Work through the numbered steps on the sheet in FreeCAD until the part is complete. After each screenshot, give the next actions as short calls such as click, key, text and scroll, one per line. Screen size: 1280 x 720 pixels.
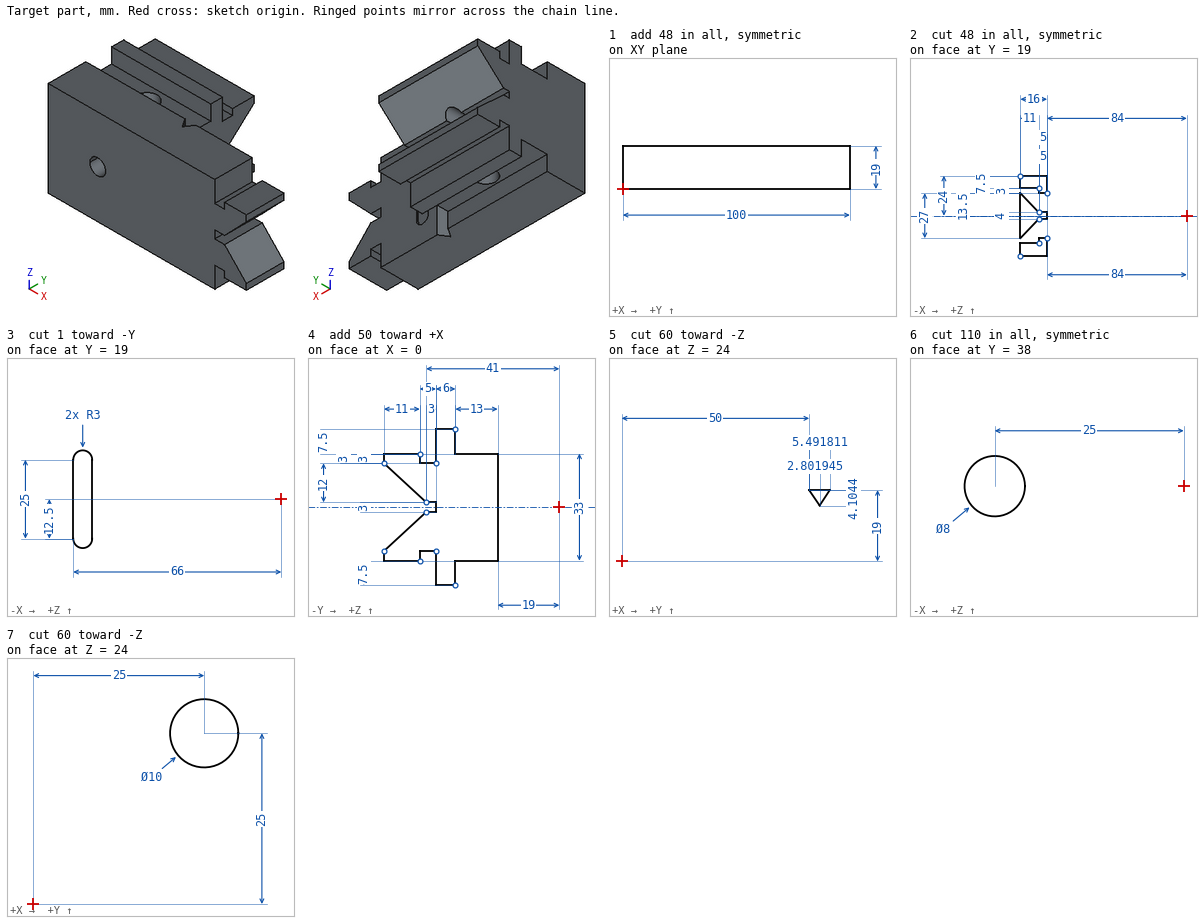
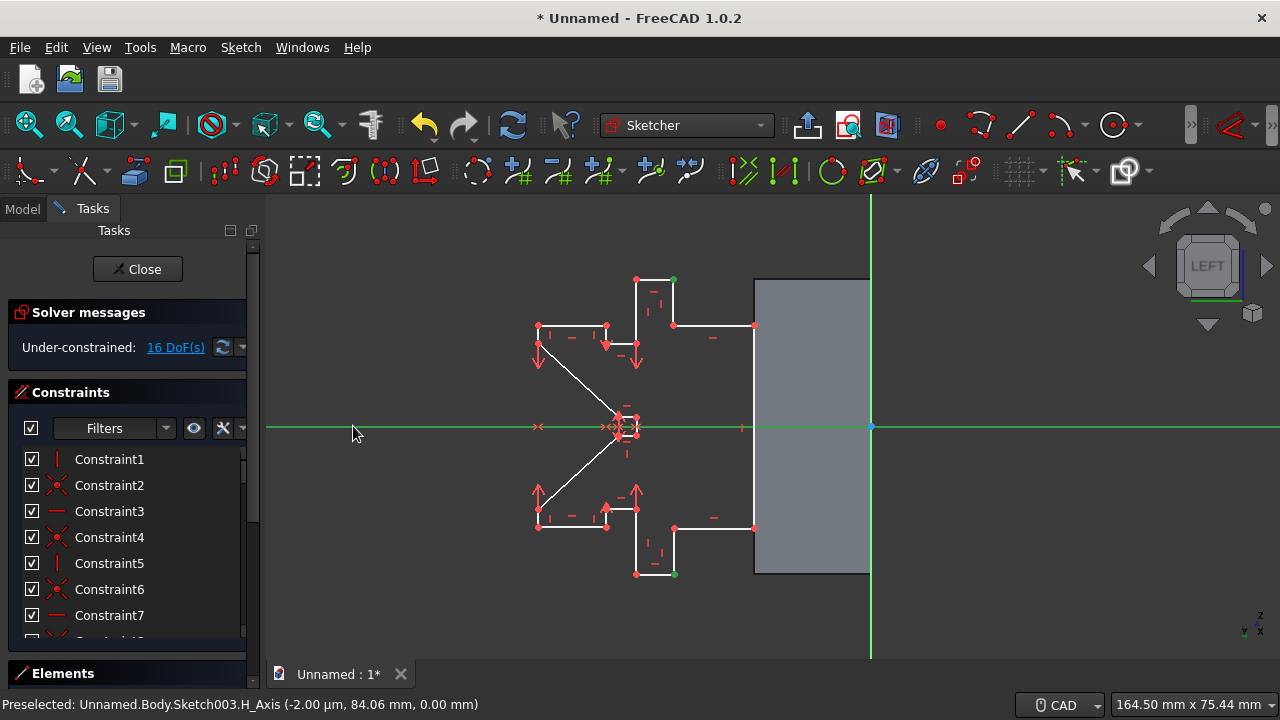
key(s)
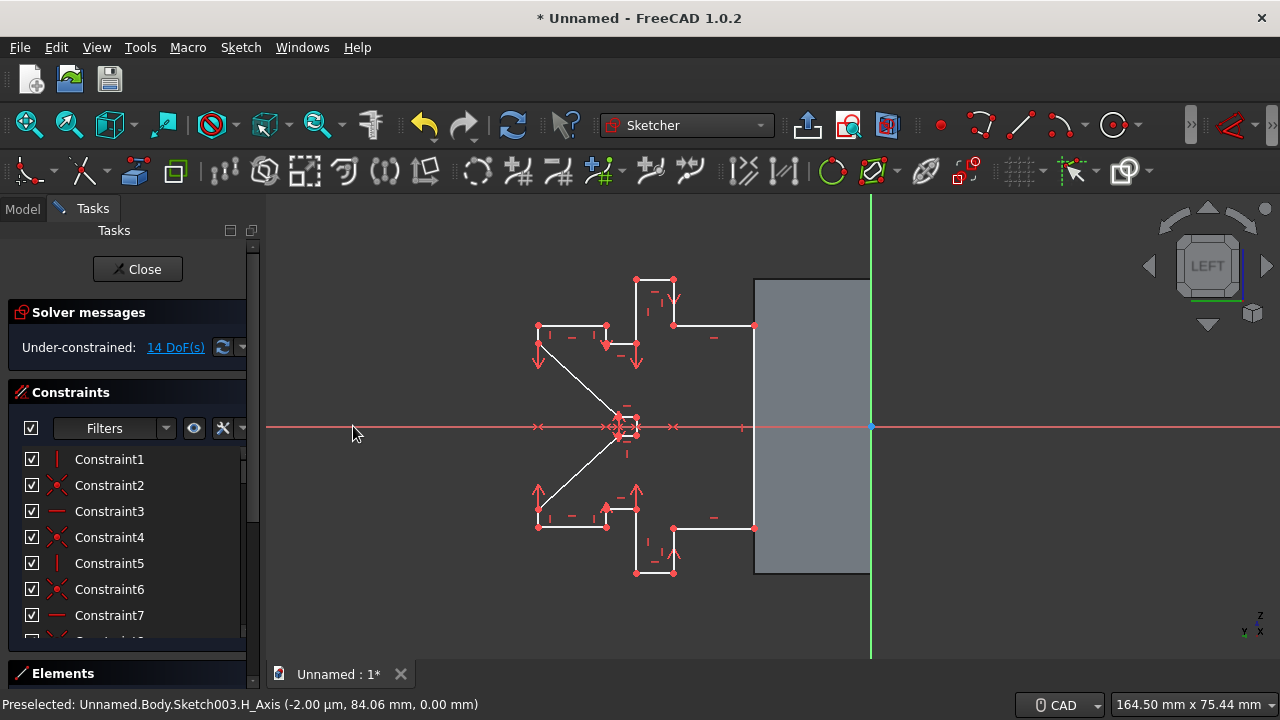
click(1230, 126)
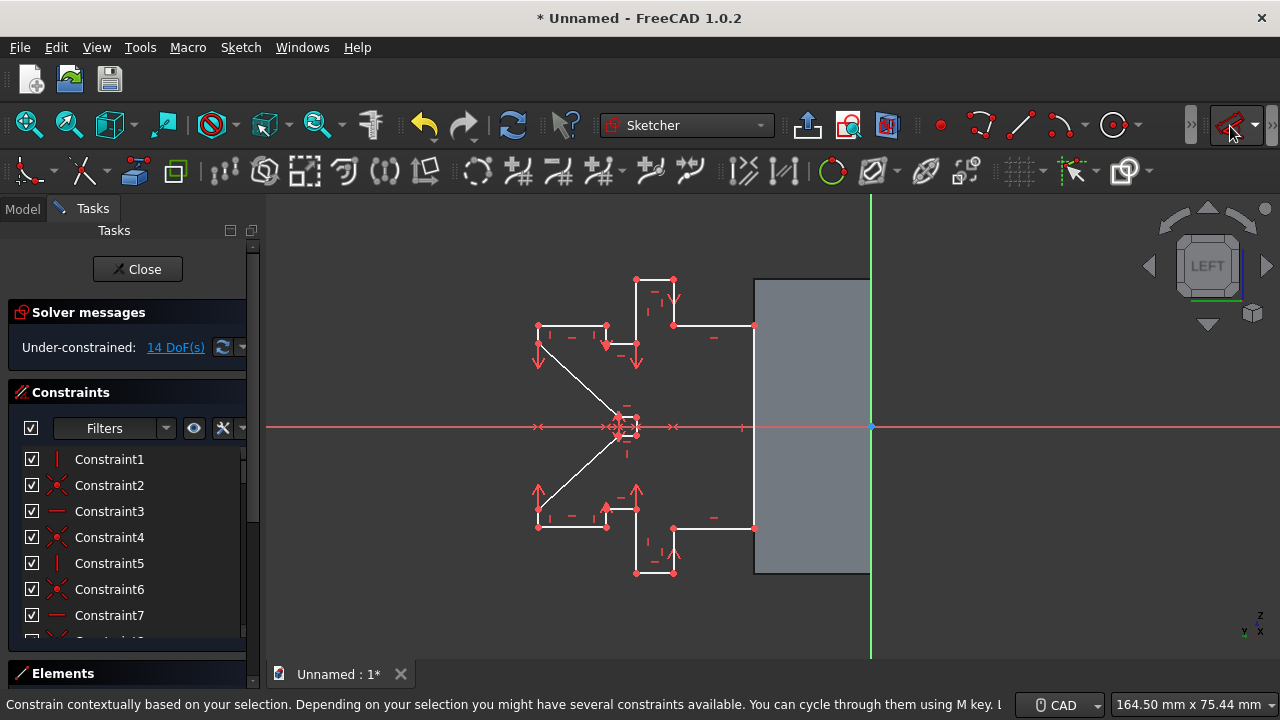
scroll(663, 280, up, 2)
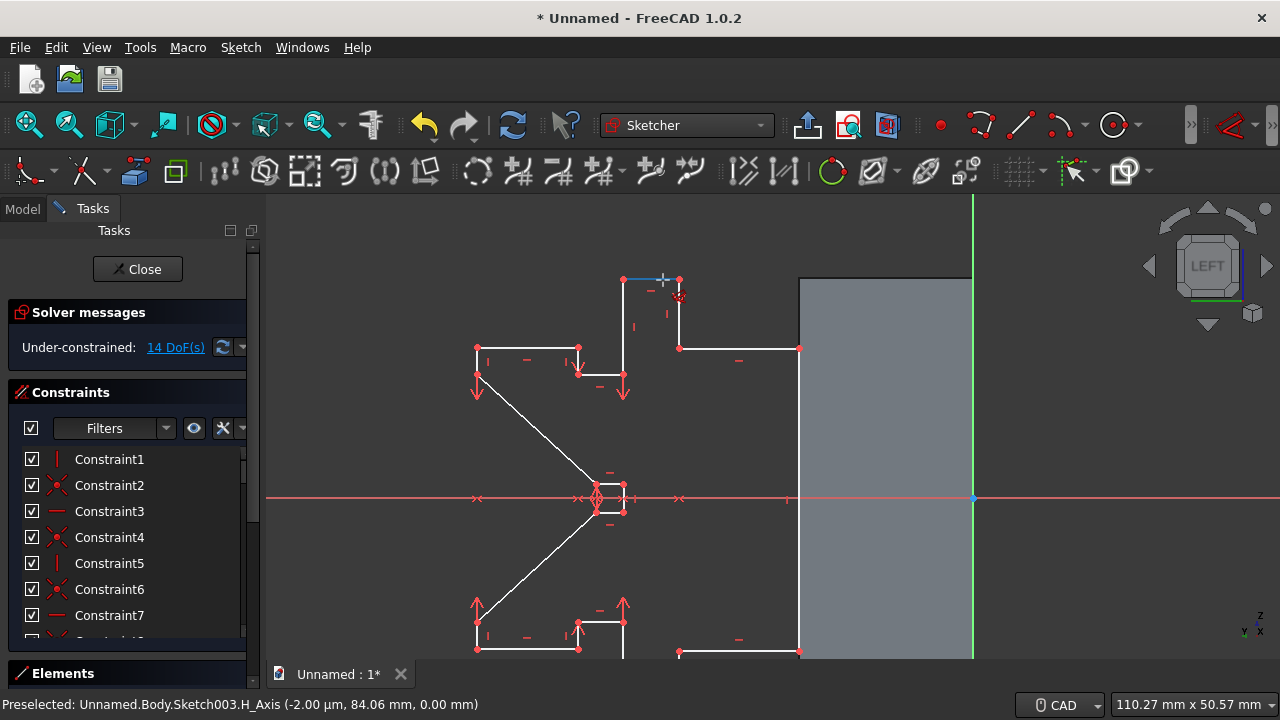
click(662, 279)
click(651, 245)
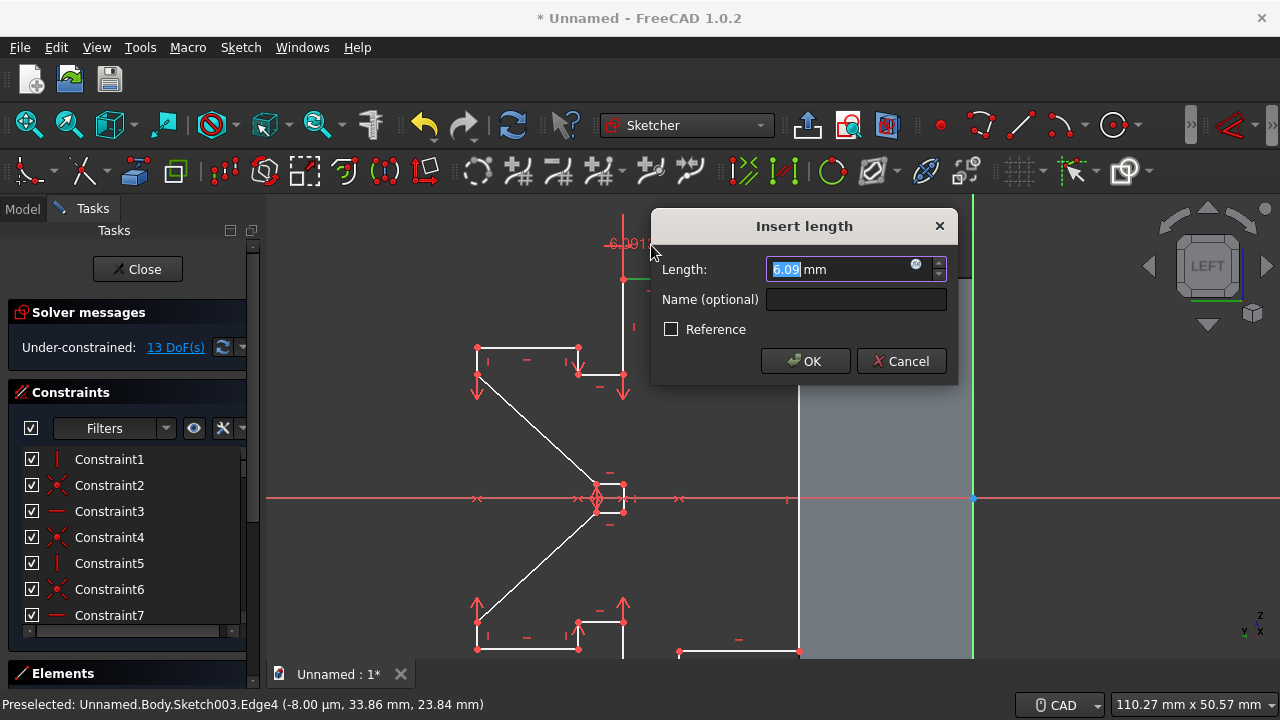
text(6)
key(Return)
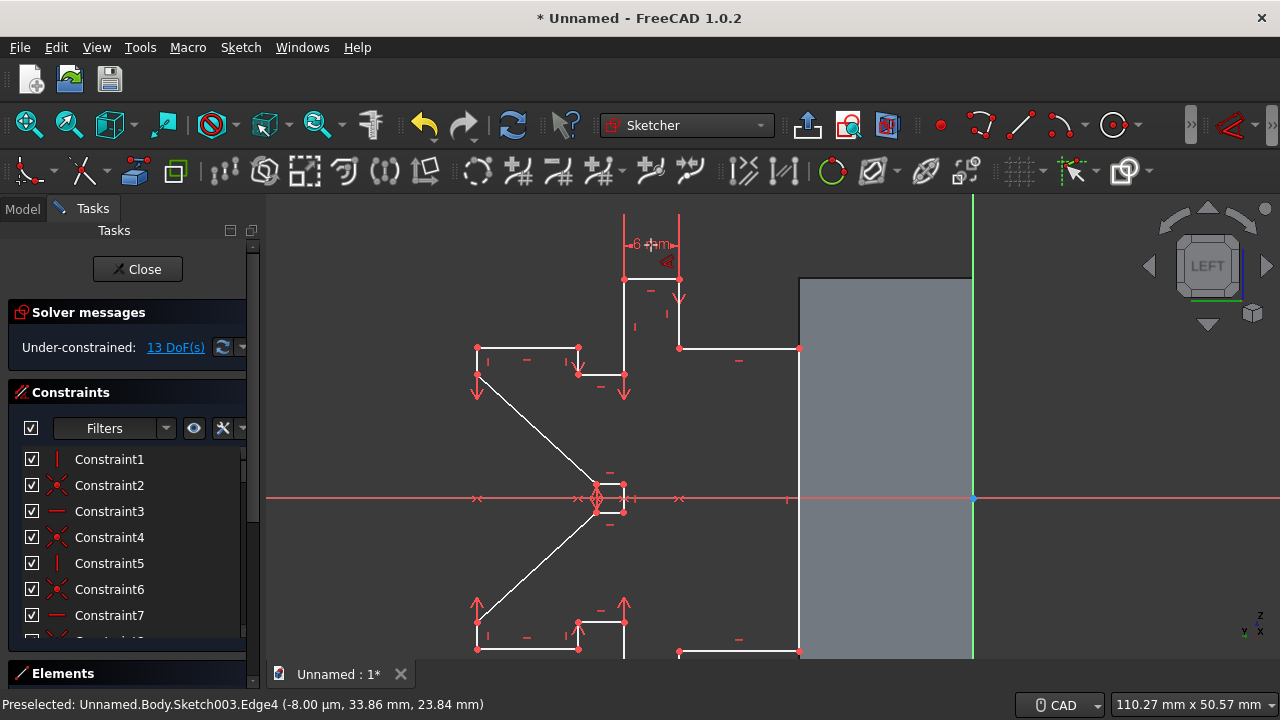
click(610, 375)
click(601, 341)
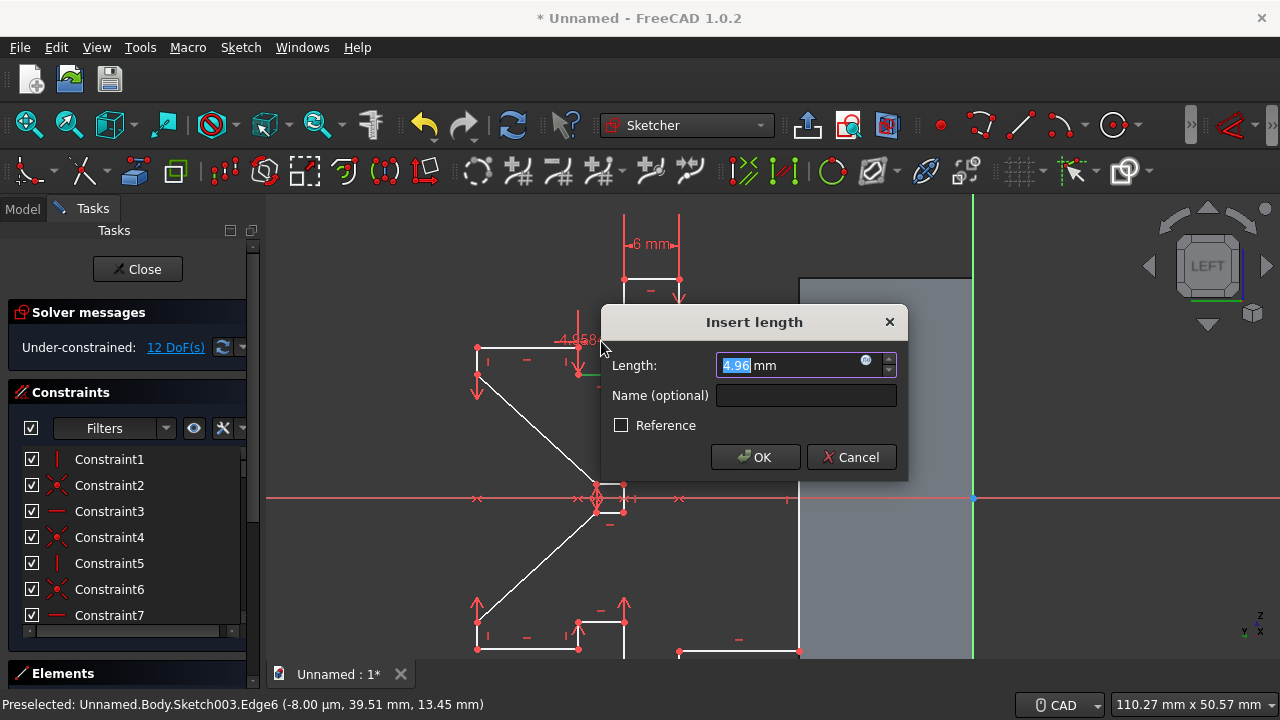
text(5)
key(Return)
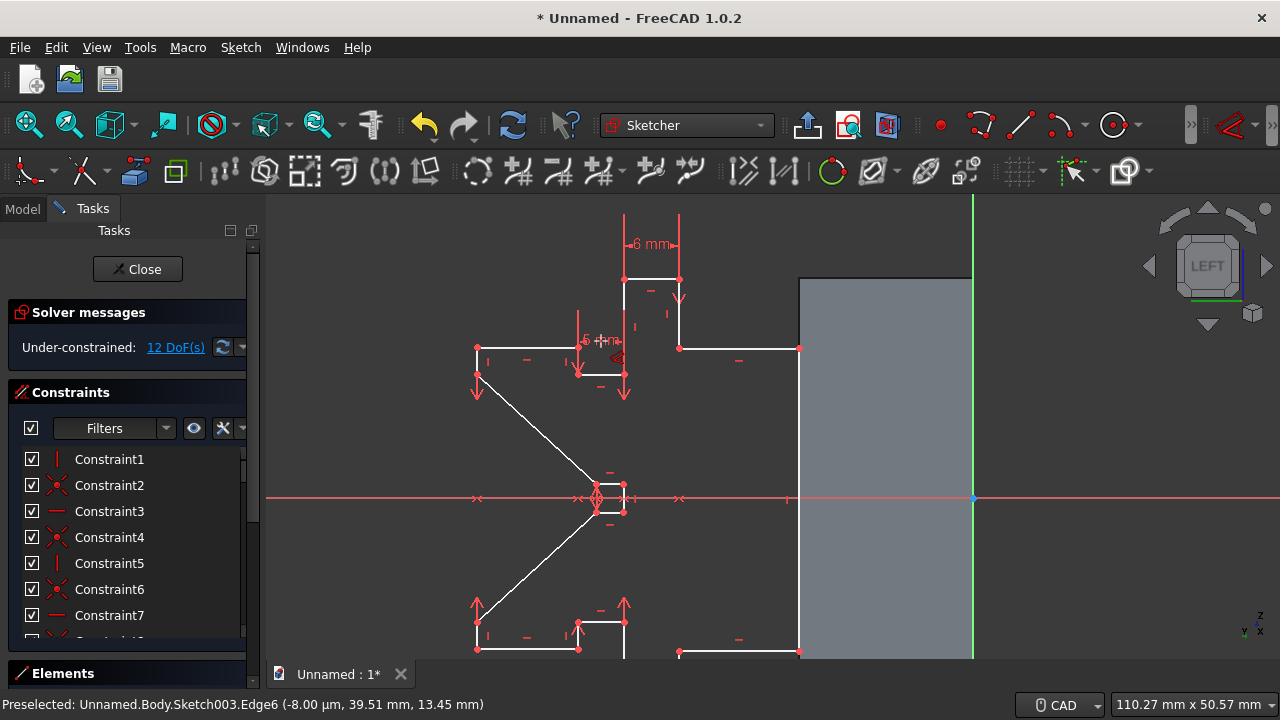
scroll(578, 364, up, 2)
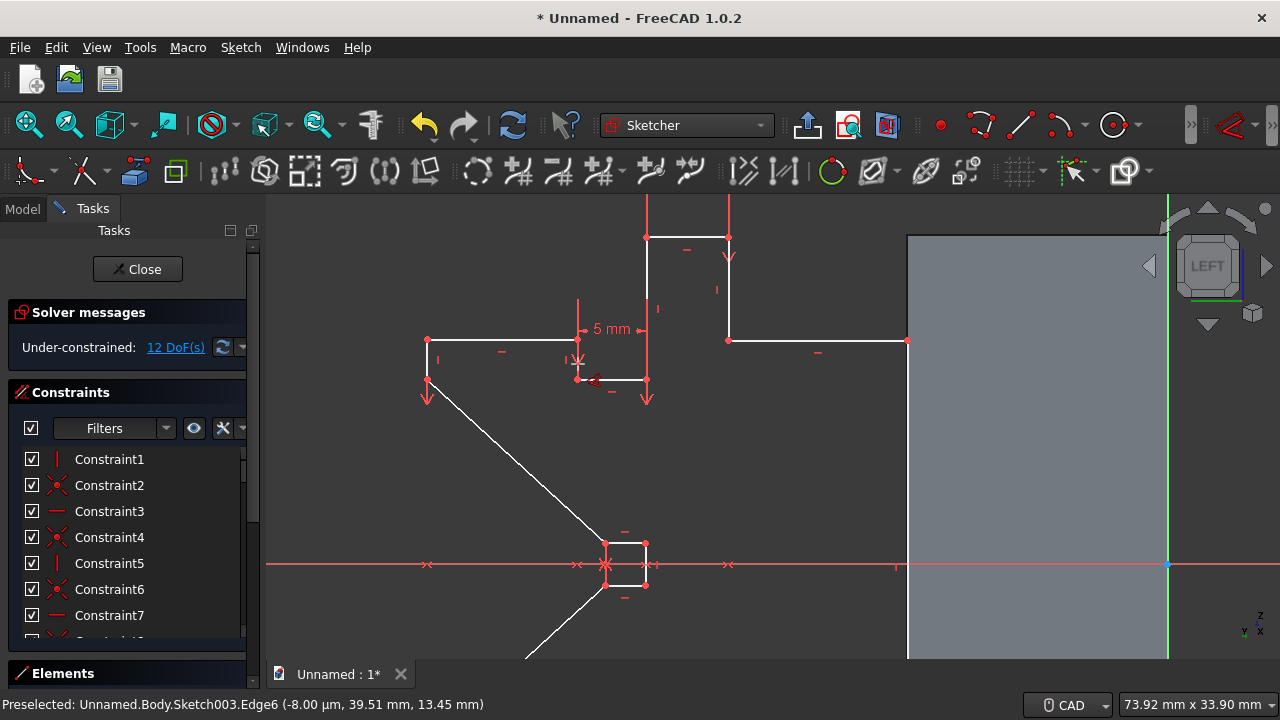
click(578, 364)
click(544, 360)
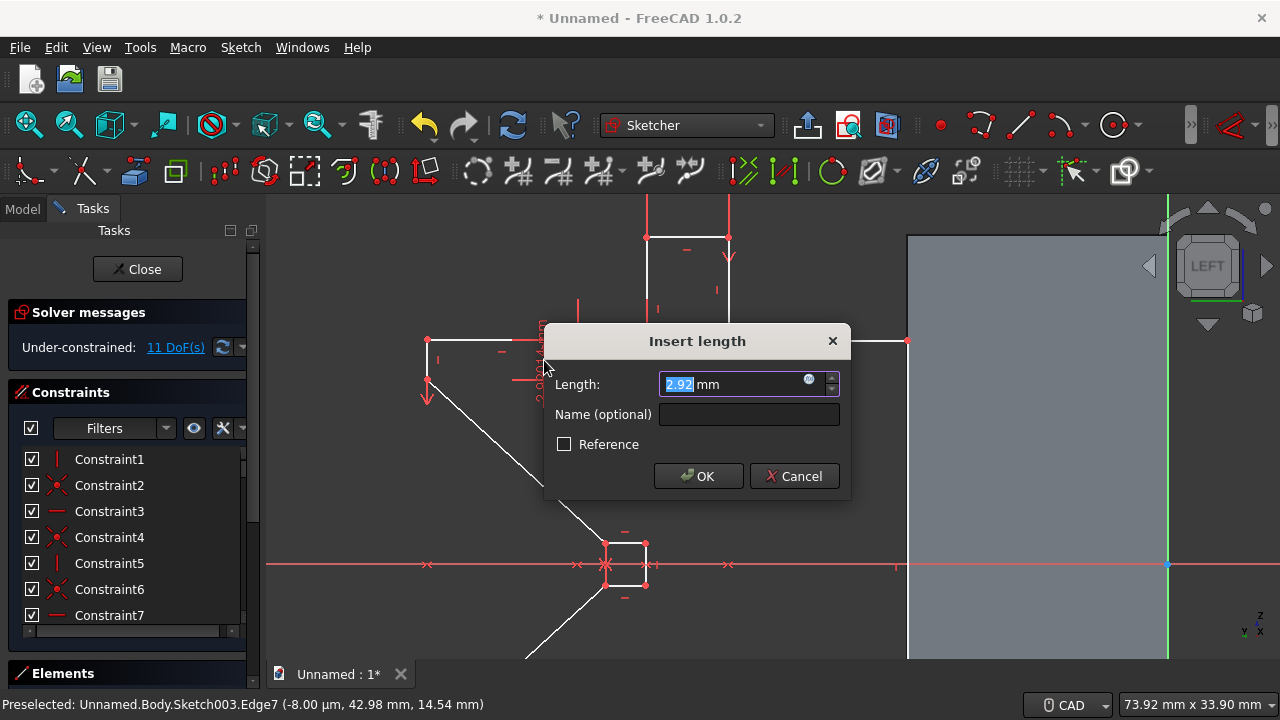
text(3)
key(Return)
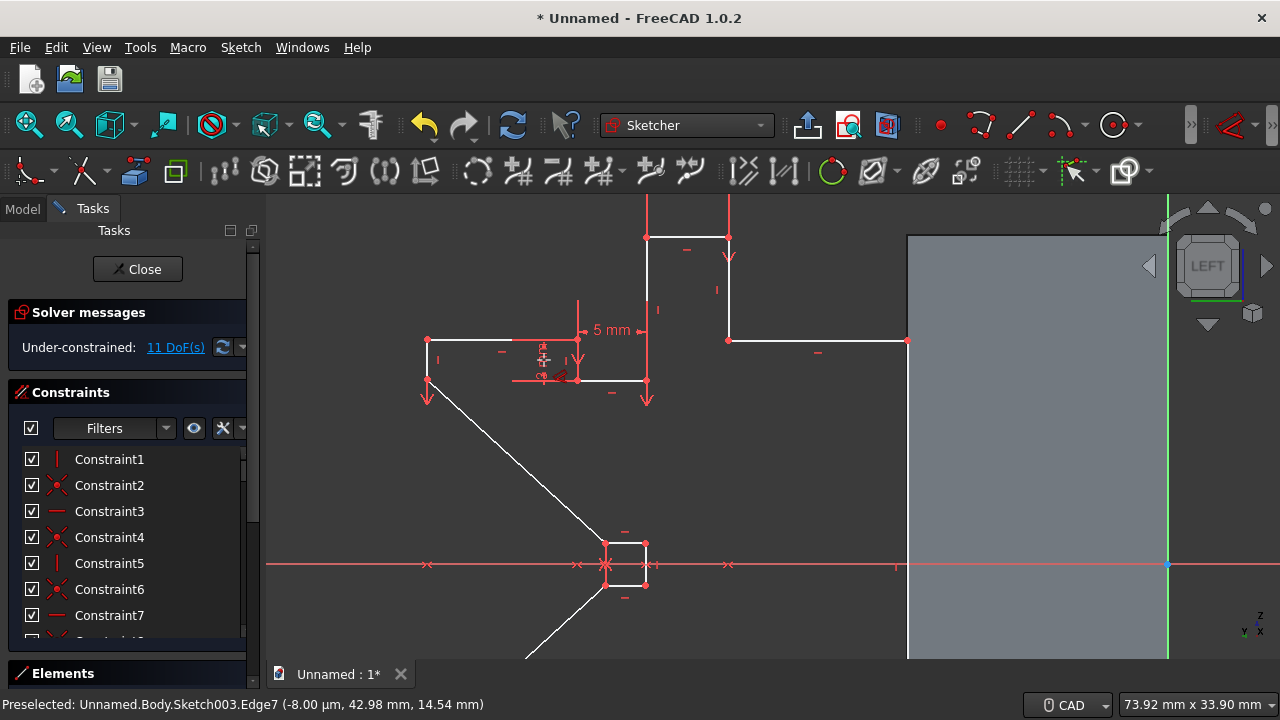
click(427, 352)
click(393, 360)